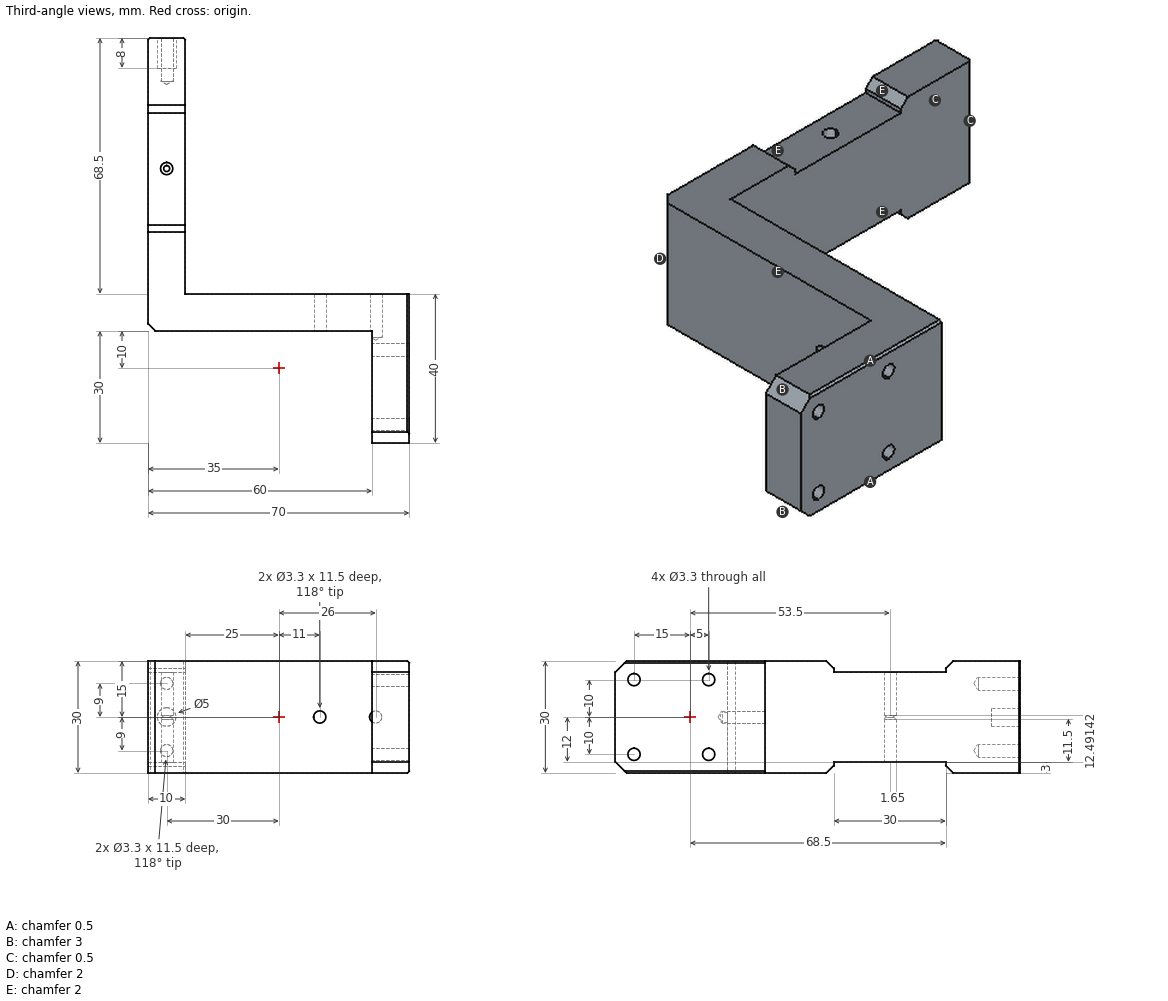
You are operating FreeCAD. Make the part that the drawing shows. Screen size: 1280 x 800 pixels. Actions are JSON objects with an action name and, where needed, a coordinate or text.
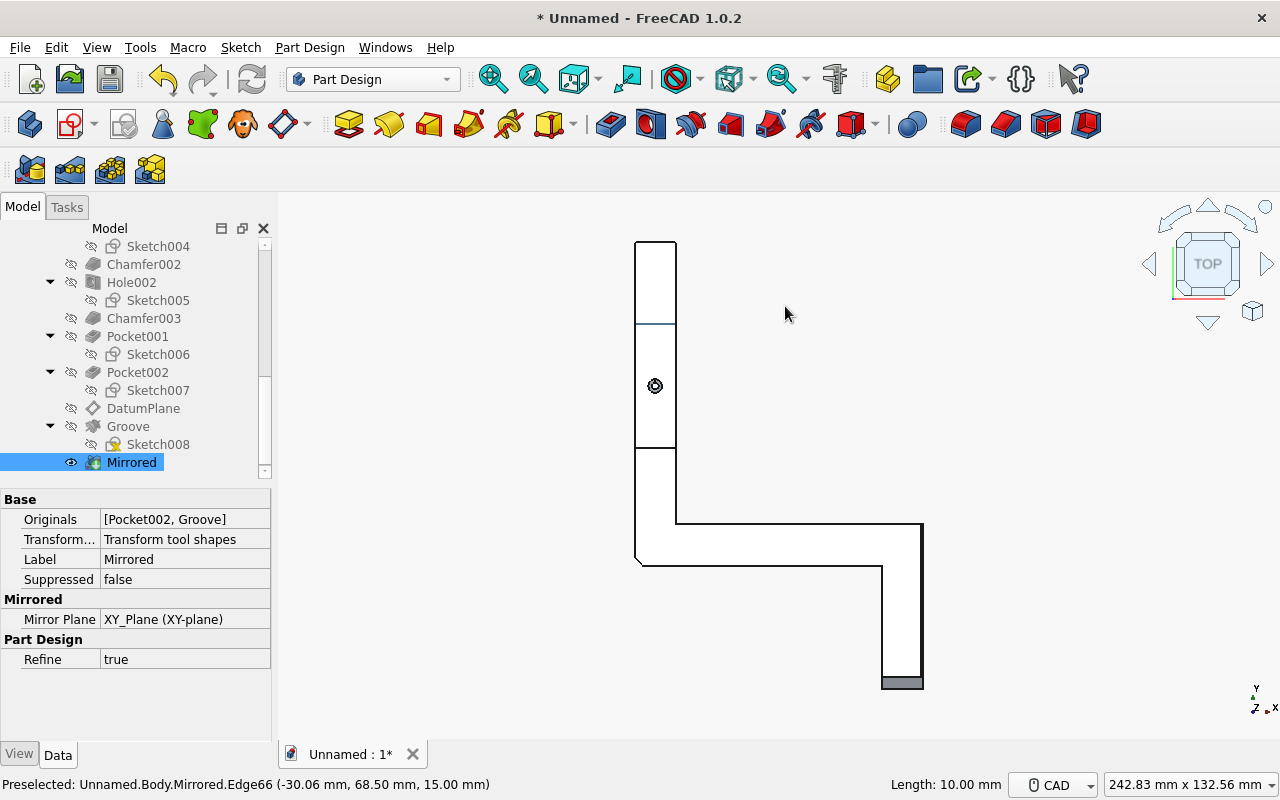
{"action": "left_click", "coordinate": [655, 447], "text": "ctrl"}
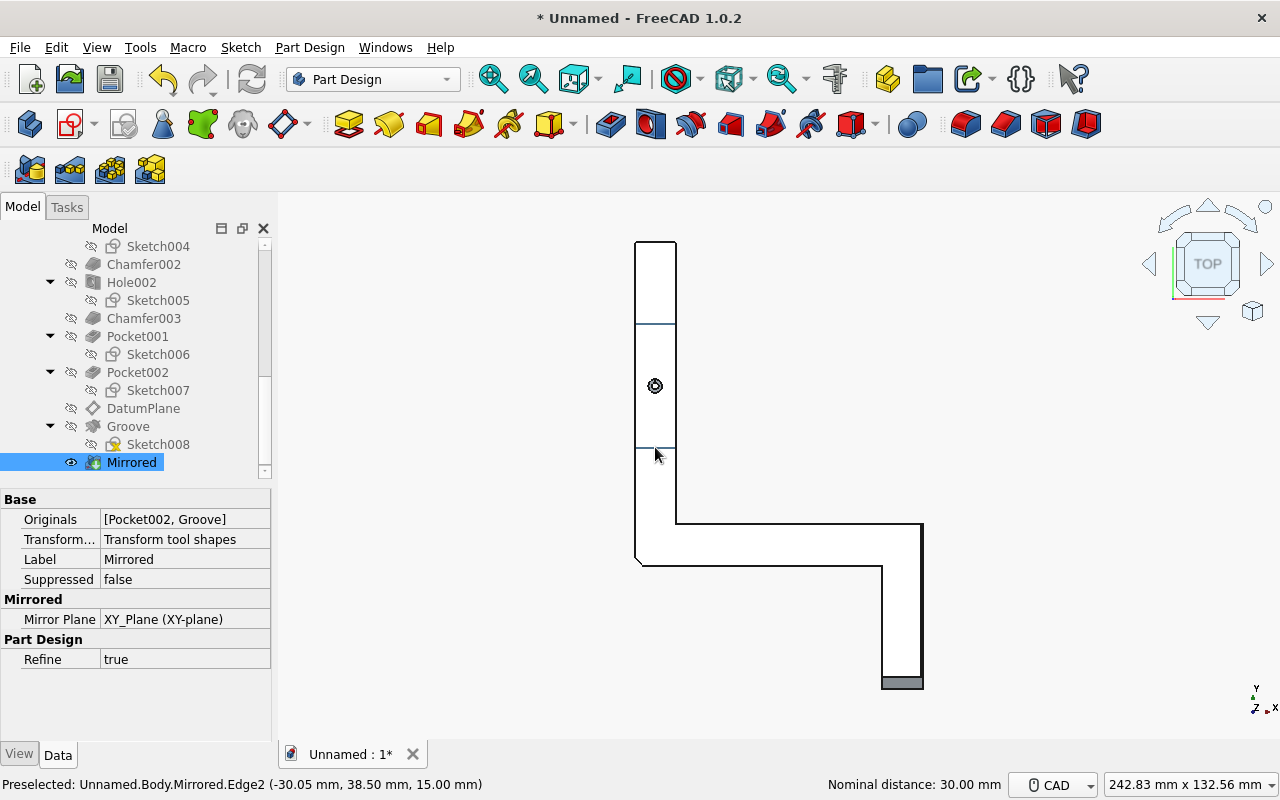
{"action": "key", "text": "1"}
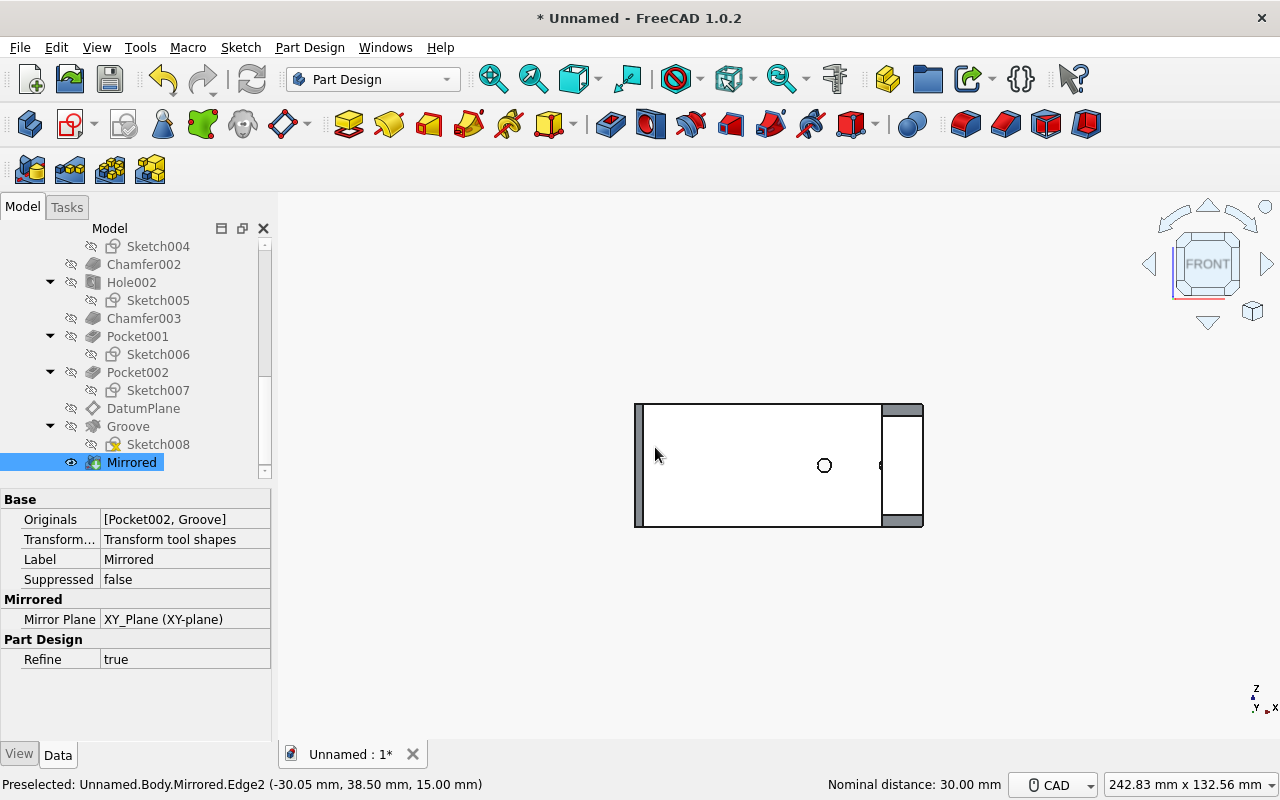
{"action": "left_click", "coordinate": [494, 80]}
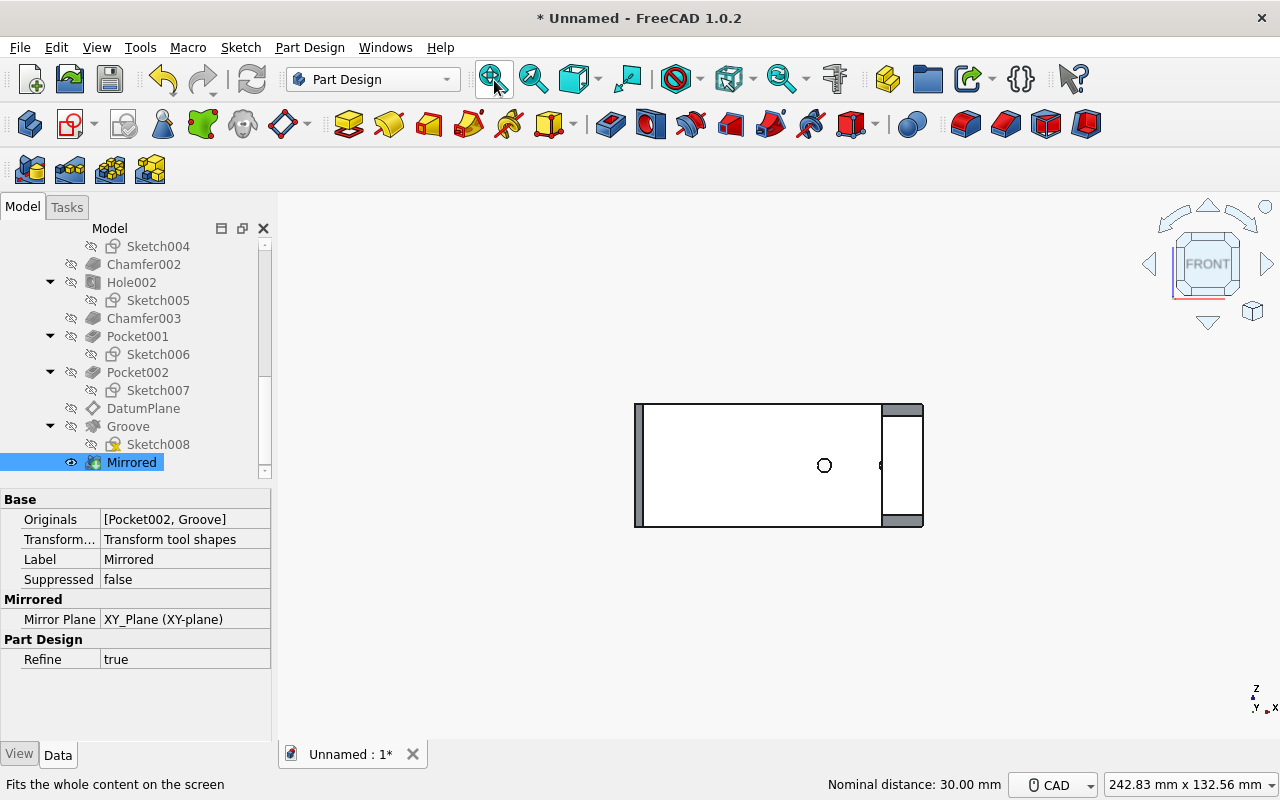
{"action": "key", "text": "3"}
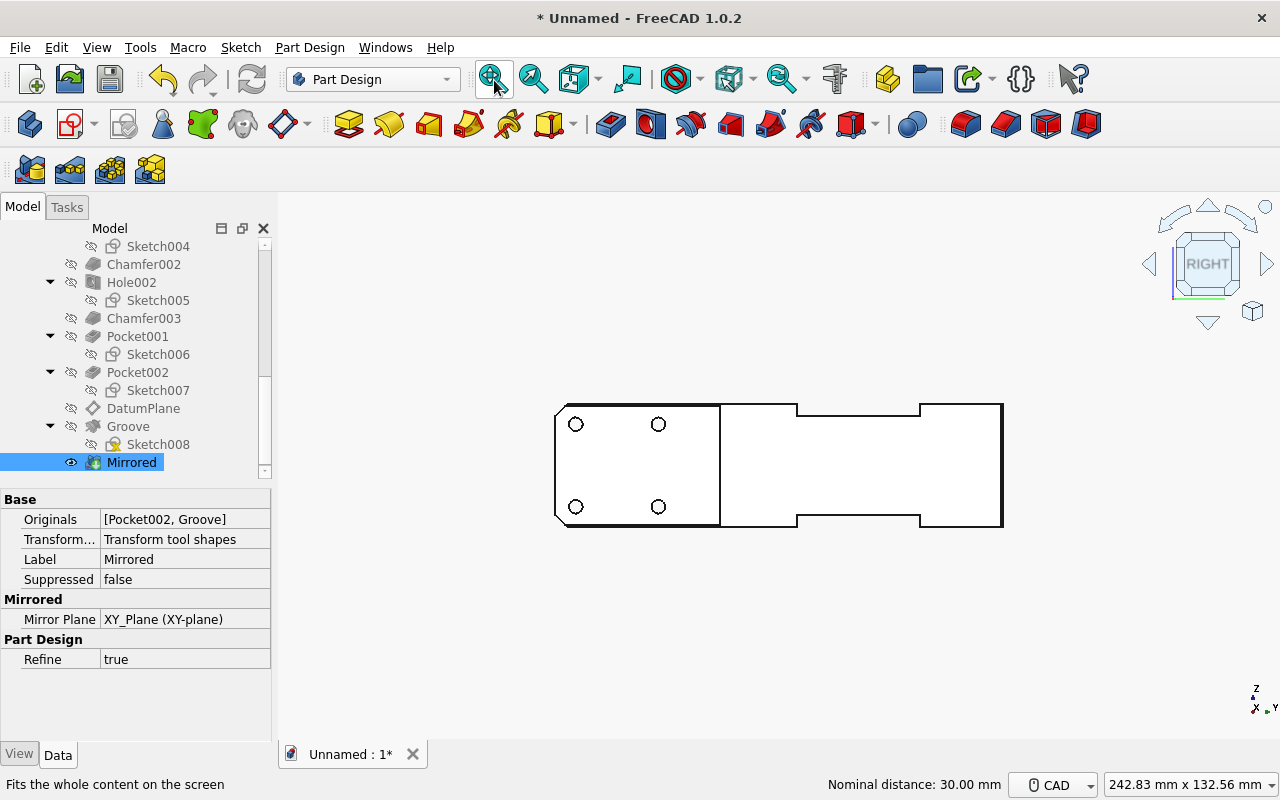
{"action": "left_click", "coordinate": [494, 80]}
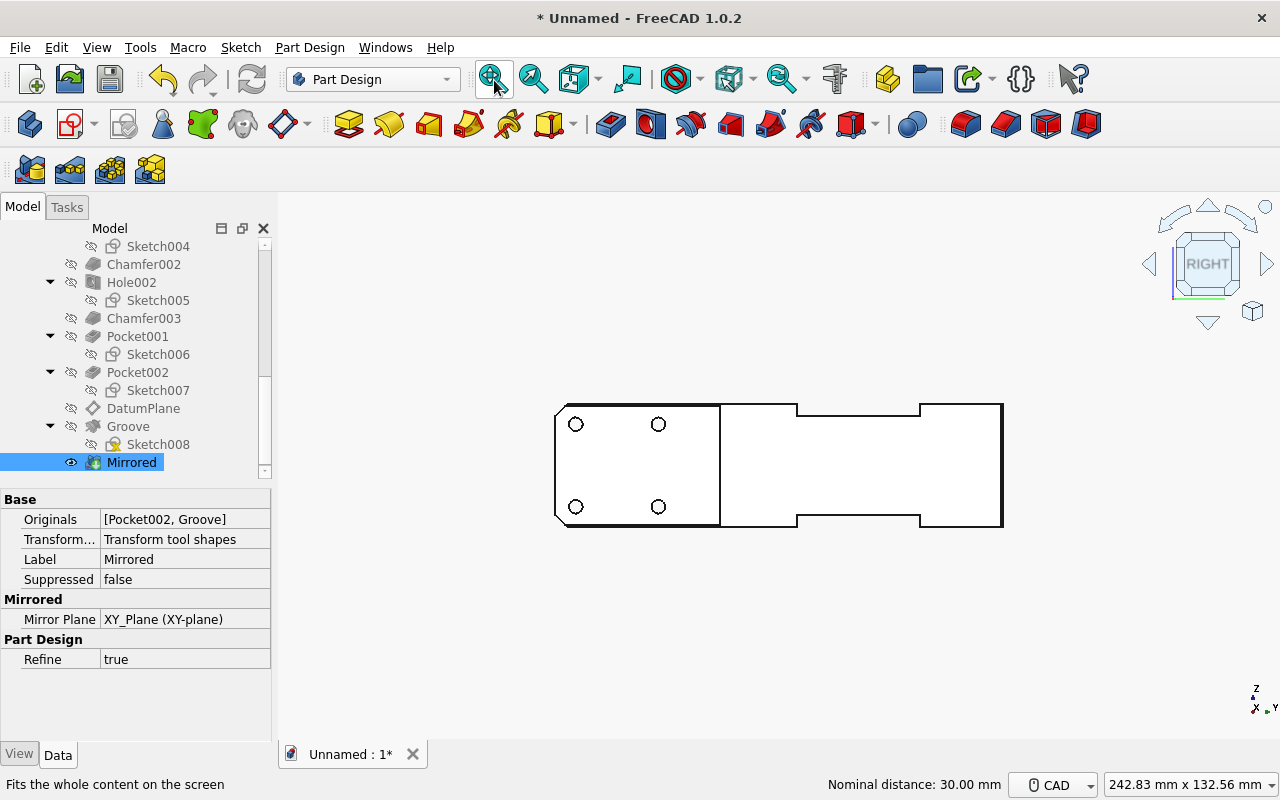
{"action": "key", "text": "5"}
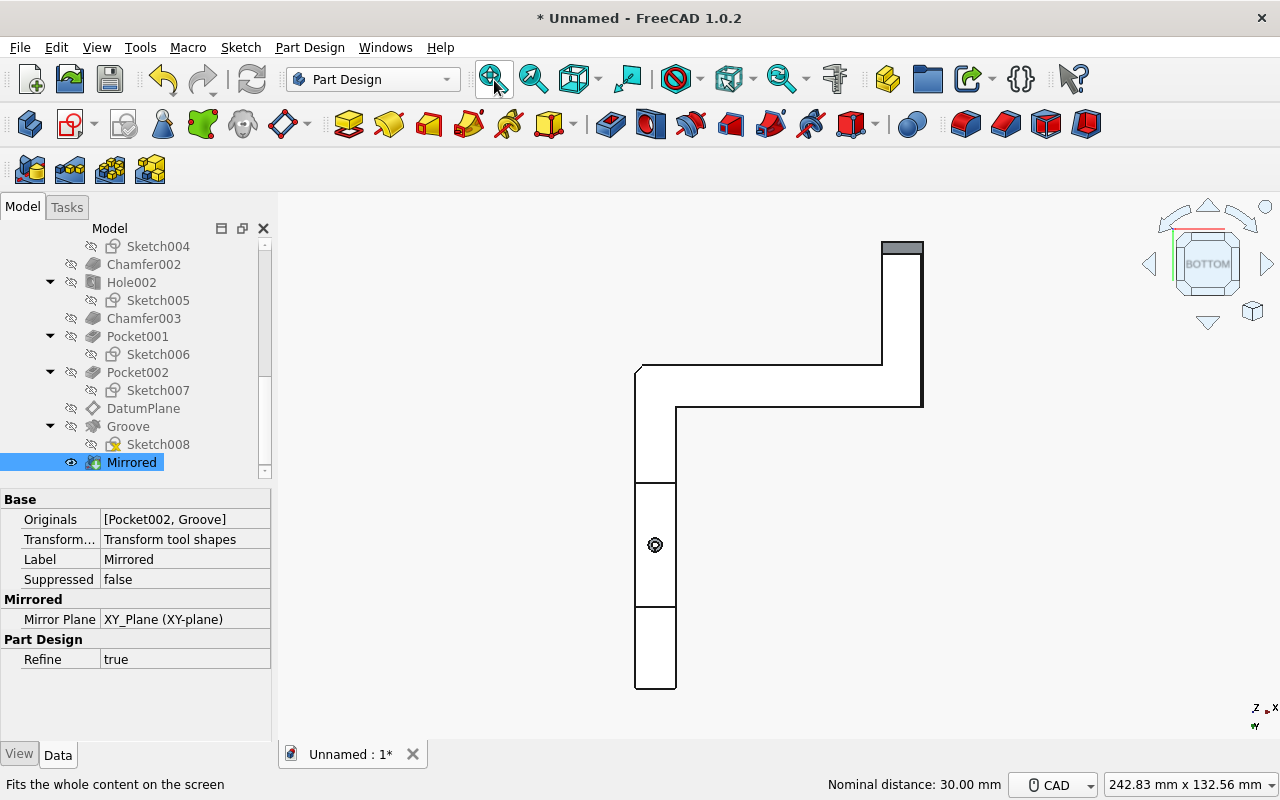
{"action": "left_click", "coordinate": [655, 482], "text": "ctrl"}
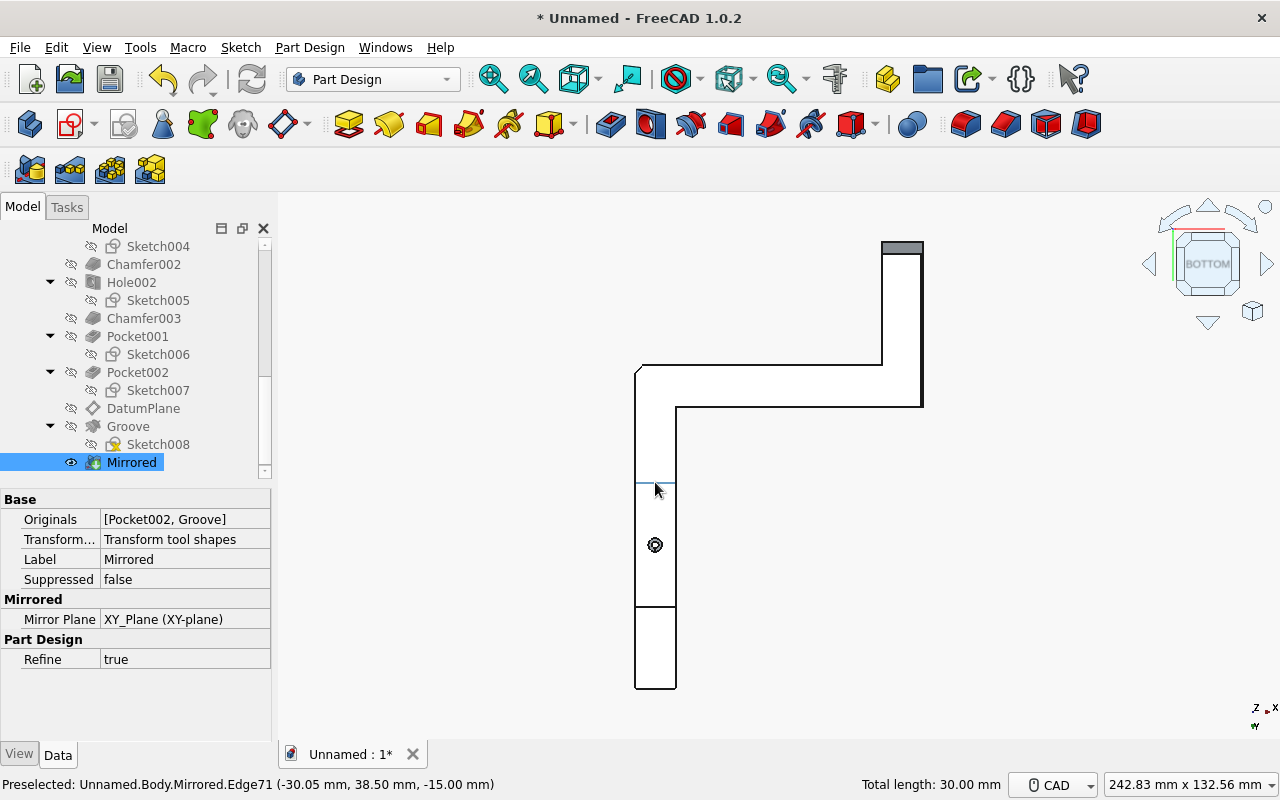
{"action": "left_click", "coordinate": [655, 606], "text": "ctrl"}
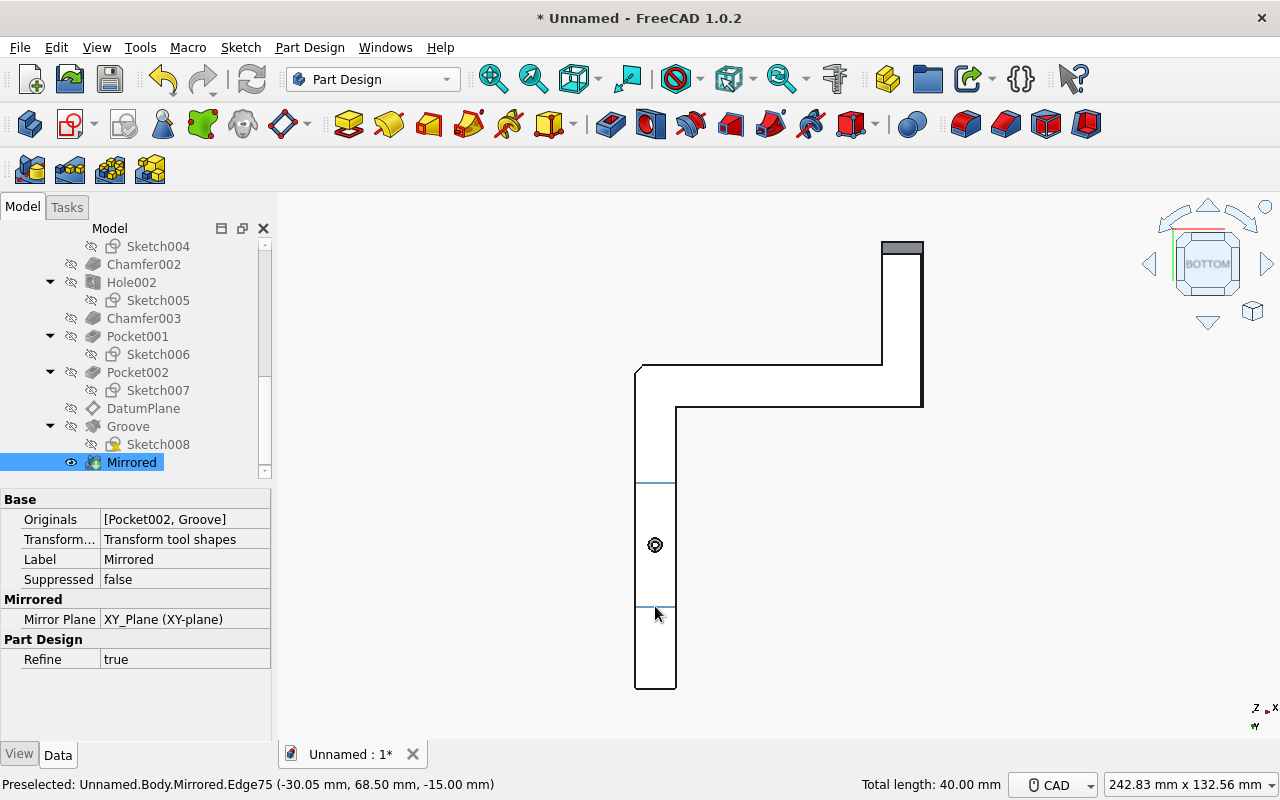
{"action": "left_click", "coordinate": [1006, 124]}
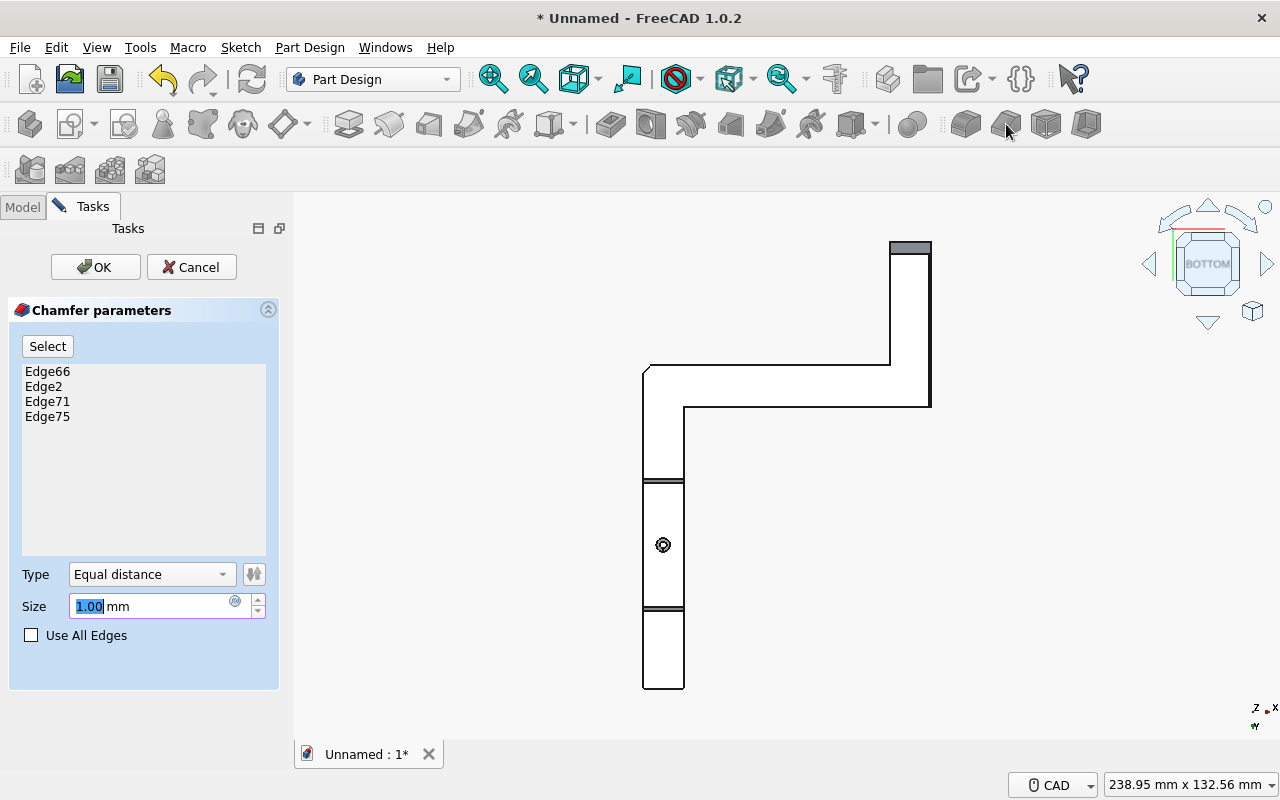
{"action": "type", "text": "2"}
{"action": "key", "text": "Tab"}